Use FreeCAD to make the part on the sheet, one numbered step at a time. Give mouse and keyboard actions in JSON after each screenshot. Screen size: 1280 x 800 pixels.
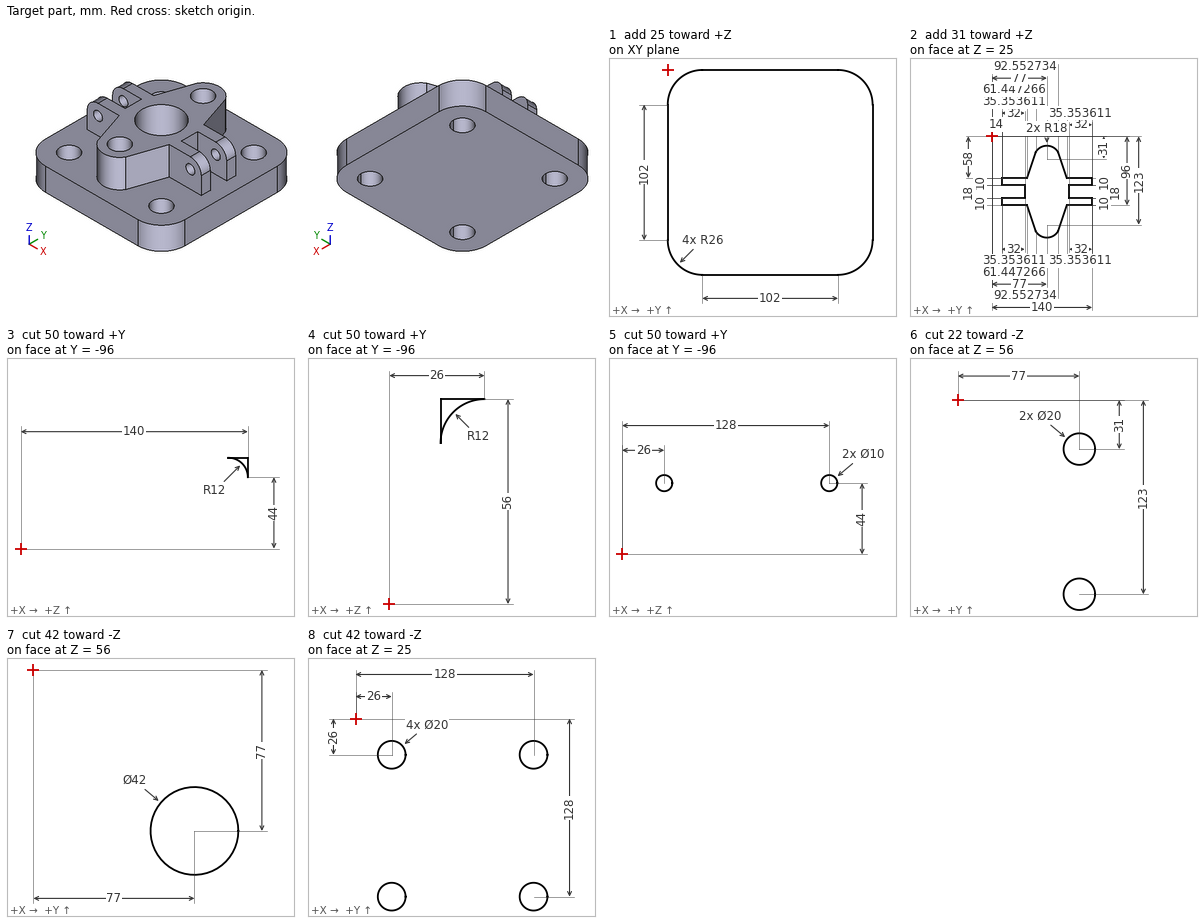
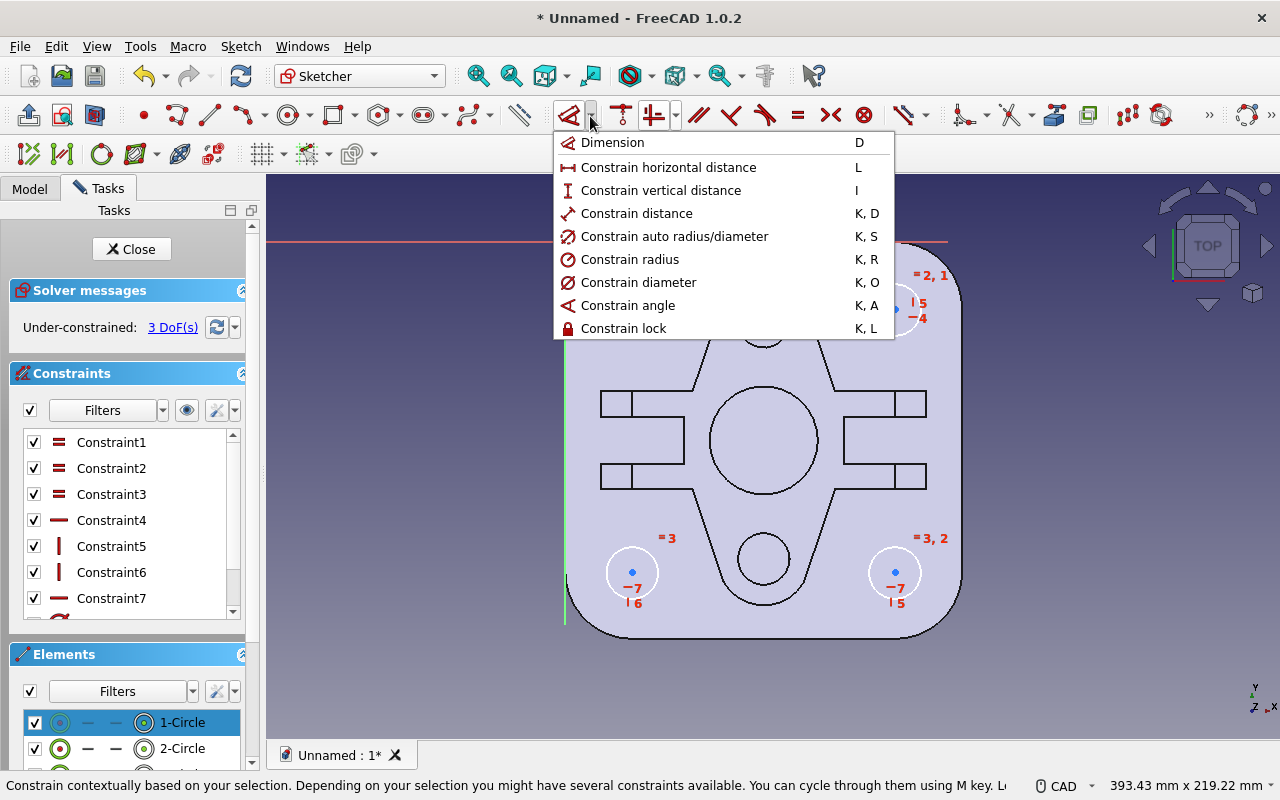
{"action": "left_click", "coordinate": [724, 190]}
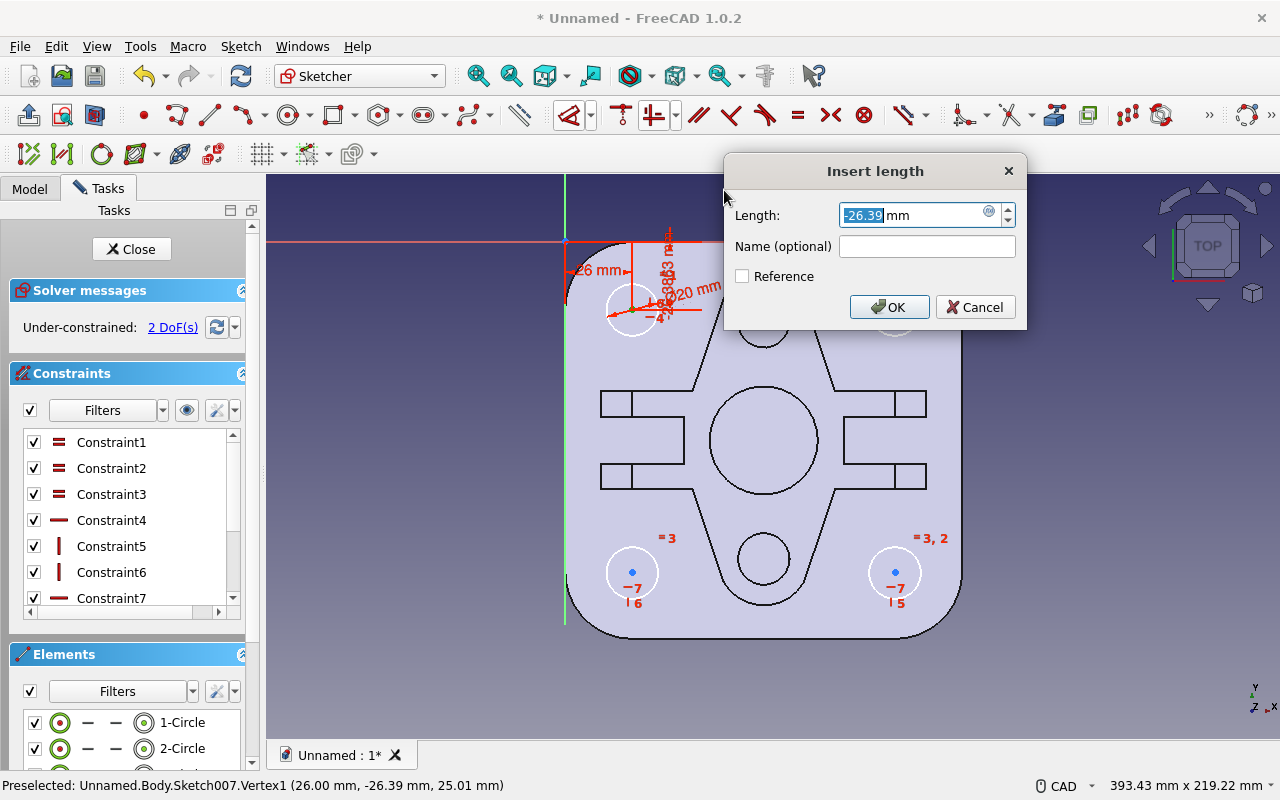
{"action": "type", "text": "-26"}
{"action": "key", "text": "Return"}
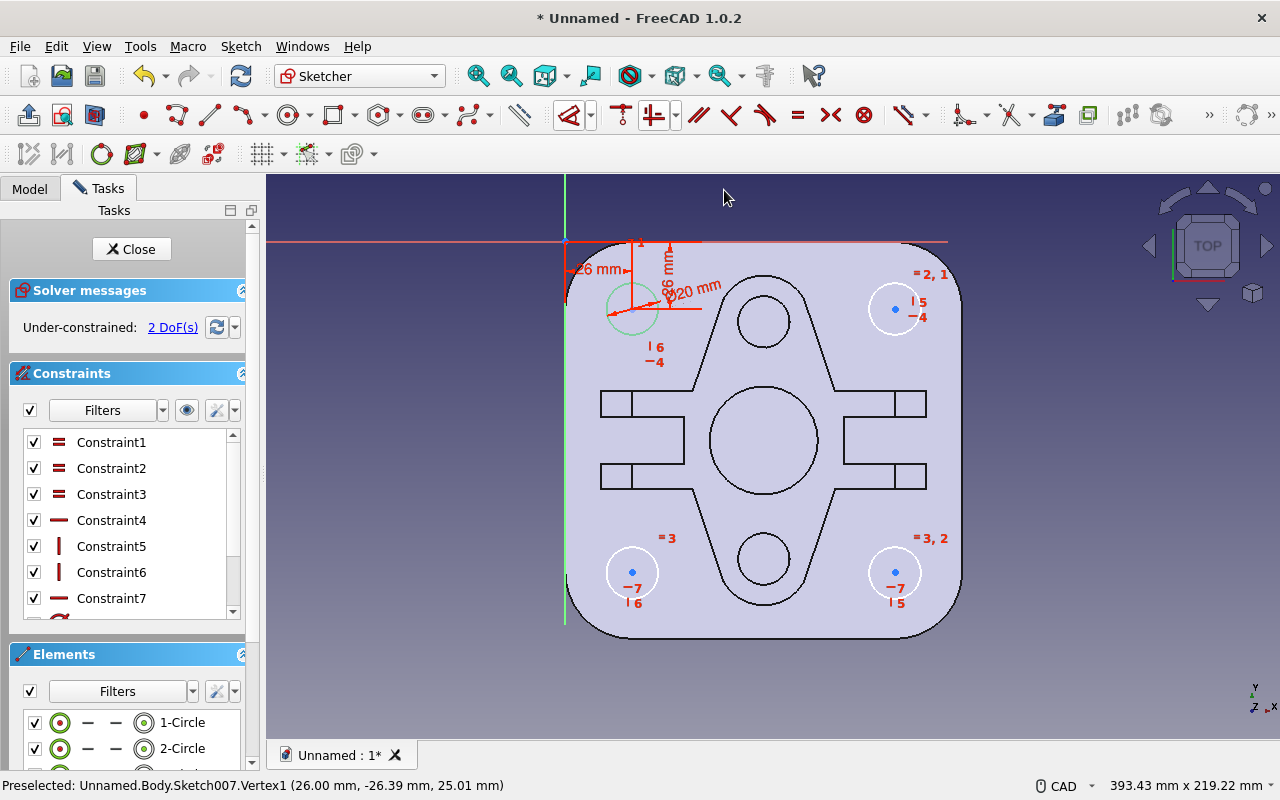
{"action": "left_click", "coordinate": [895, 309]}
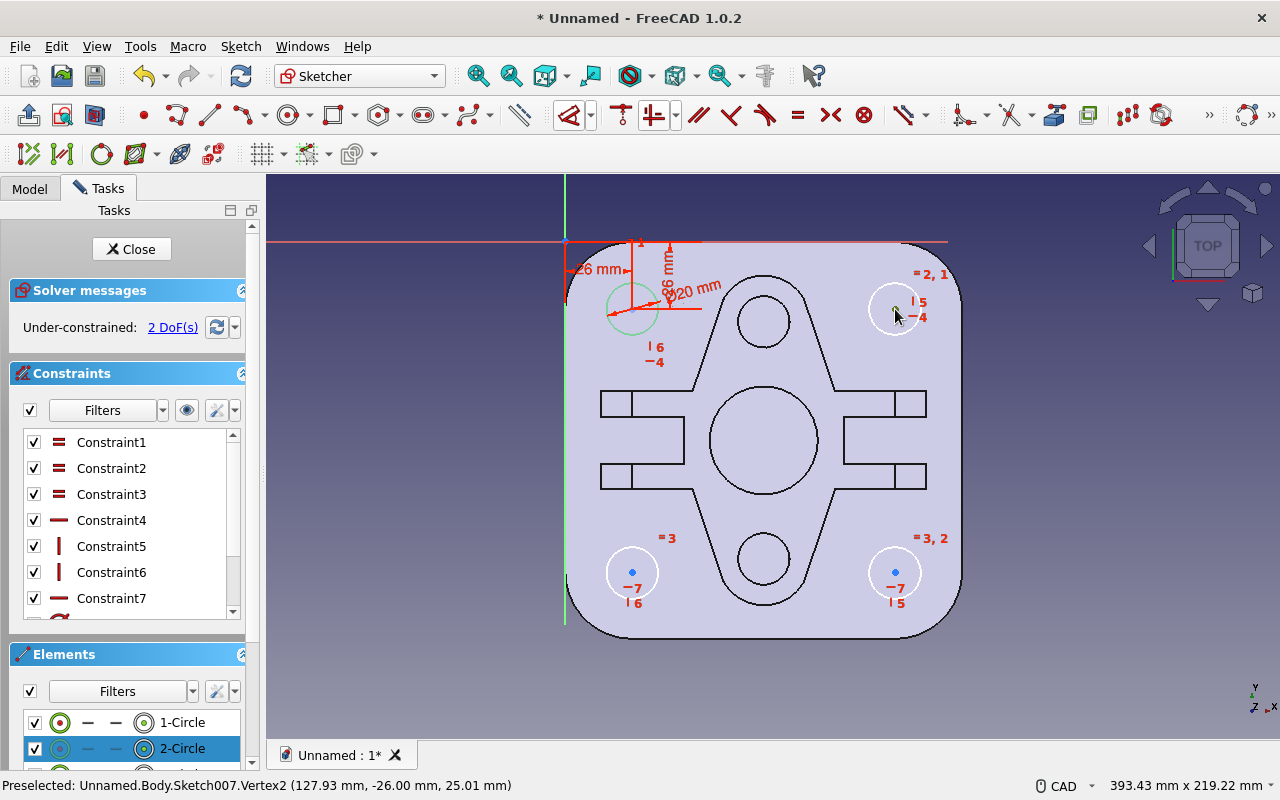
{"action": "key", "text": "l"}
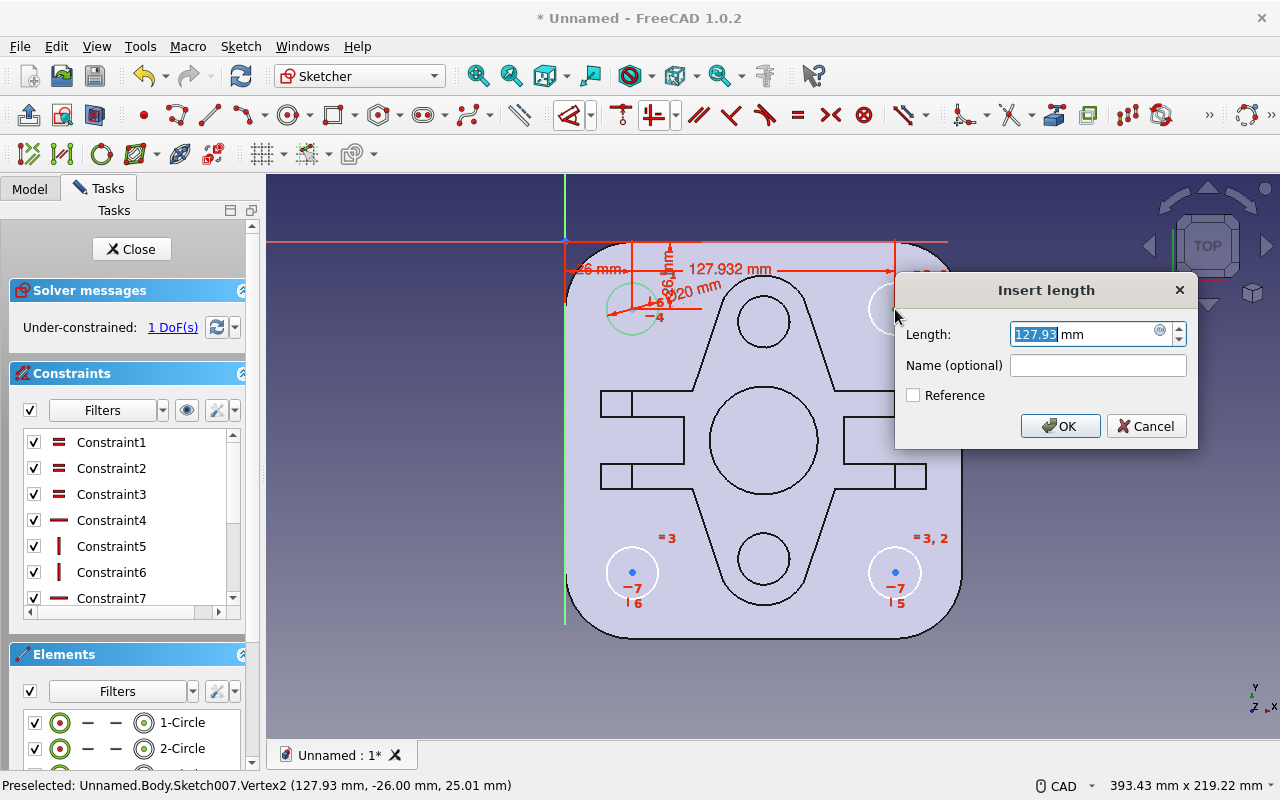
{"action": "type", "text": "128"}
{"action": "key", "text": "Return"}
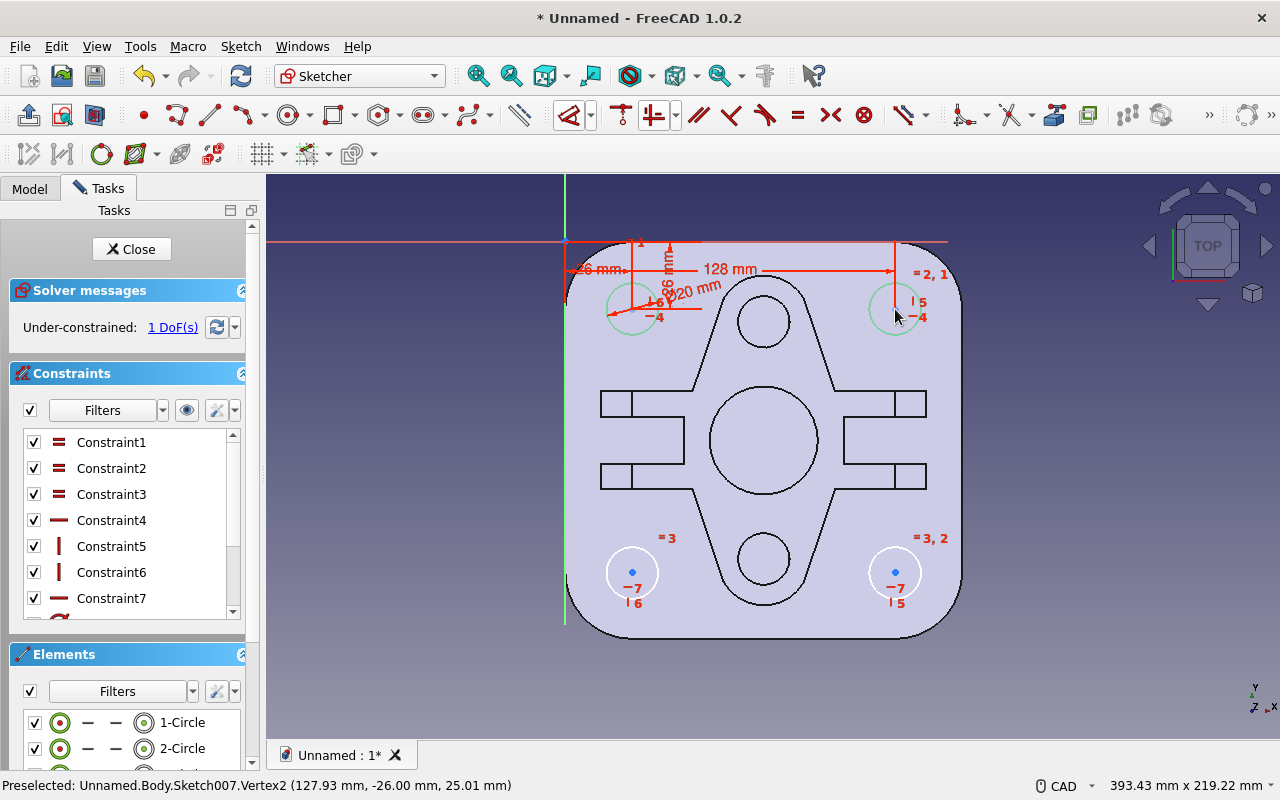
{"action": "left_click", "coordinate": [895, 573]}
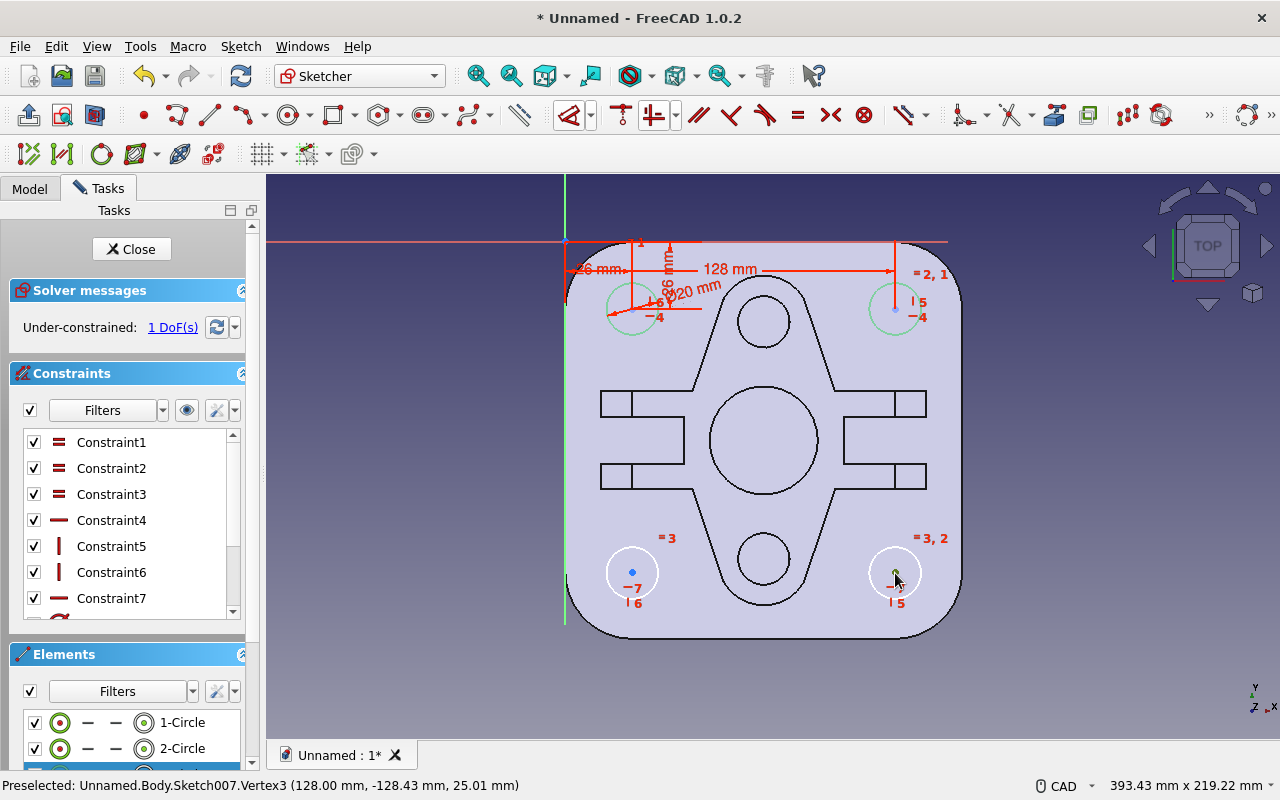
{"action": "left_click", "coordinate": [590, 116]}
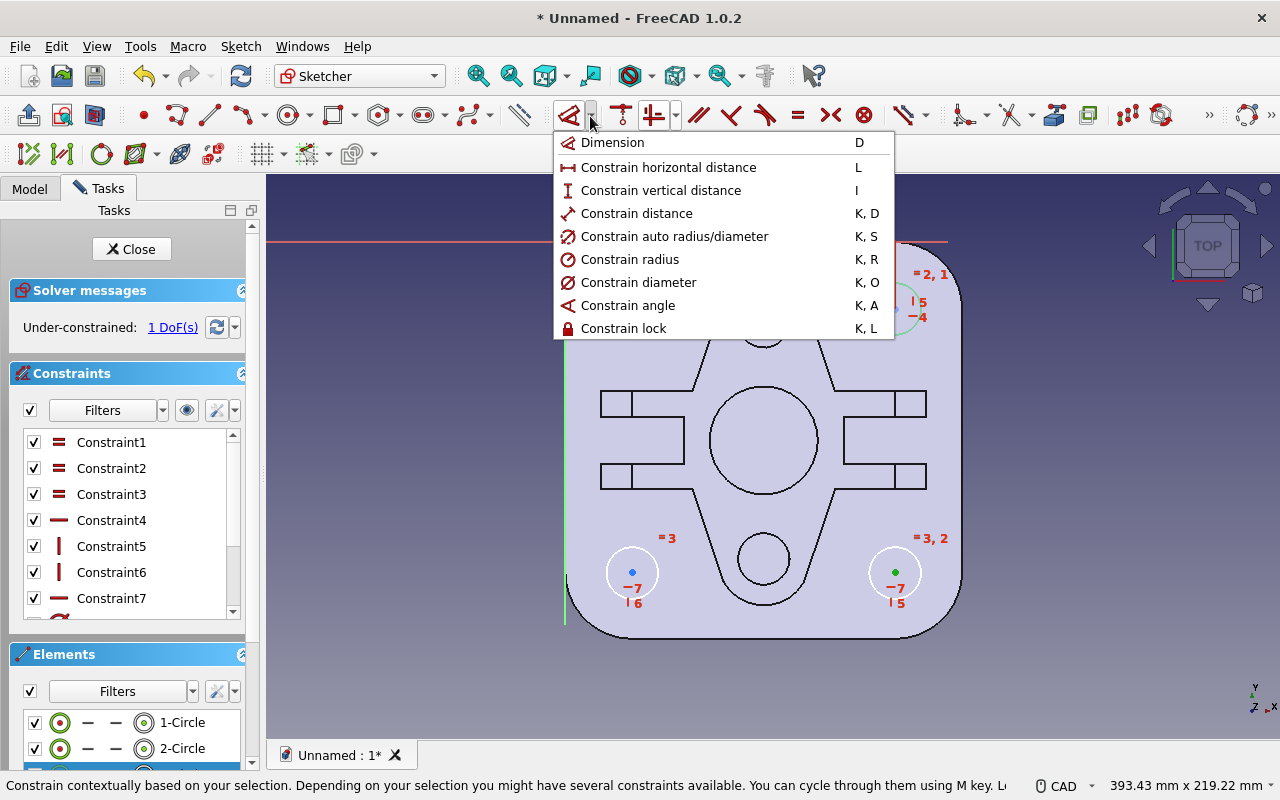
{"action": "left_click", "coordinate": [724, 190]}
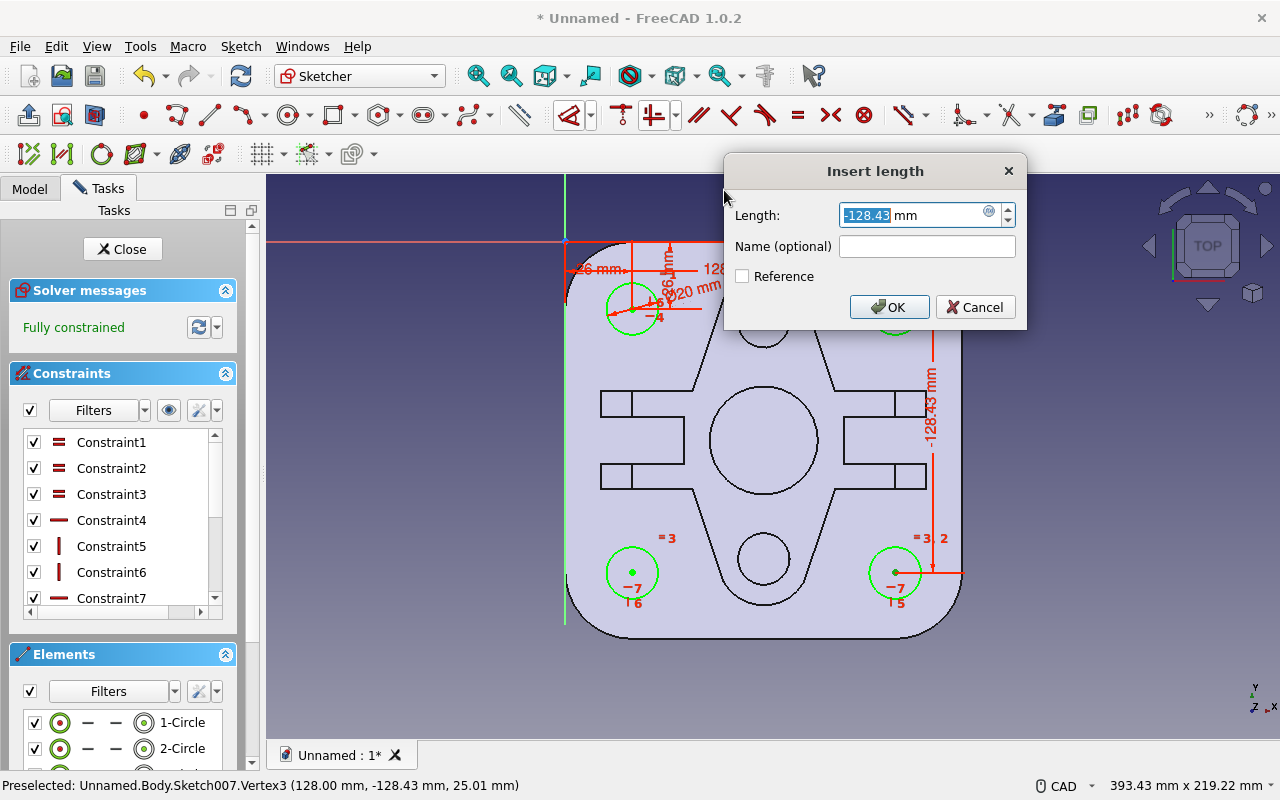
{"action": "type", "text": "-128"}
{"action": "key", "text": "Return"}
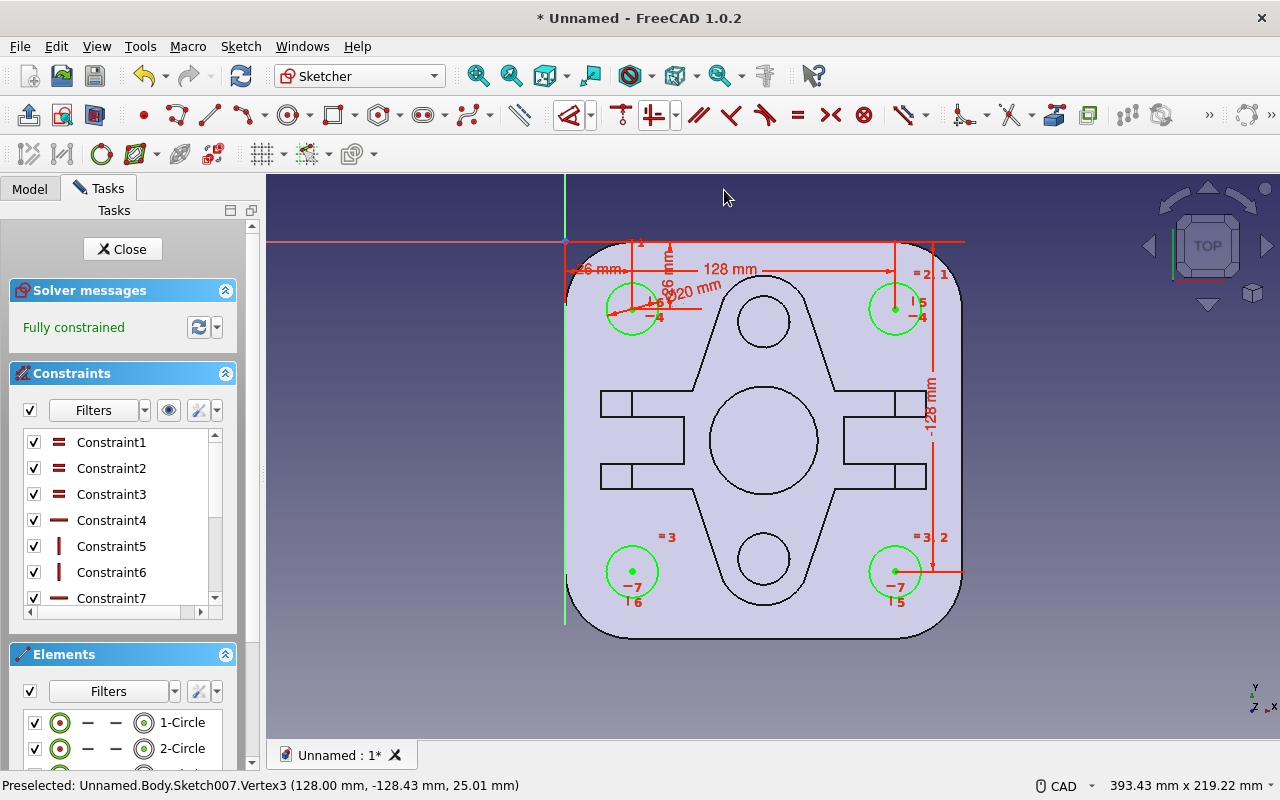
{"action": "left_click", "coordinate": [123, 249]}